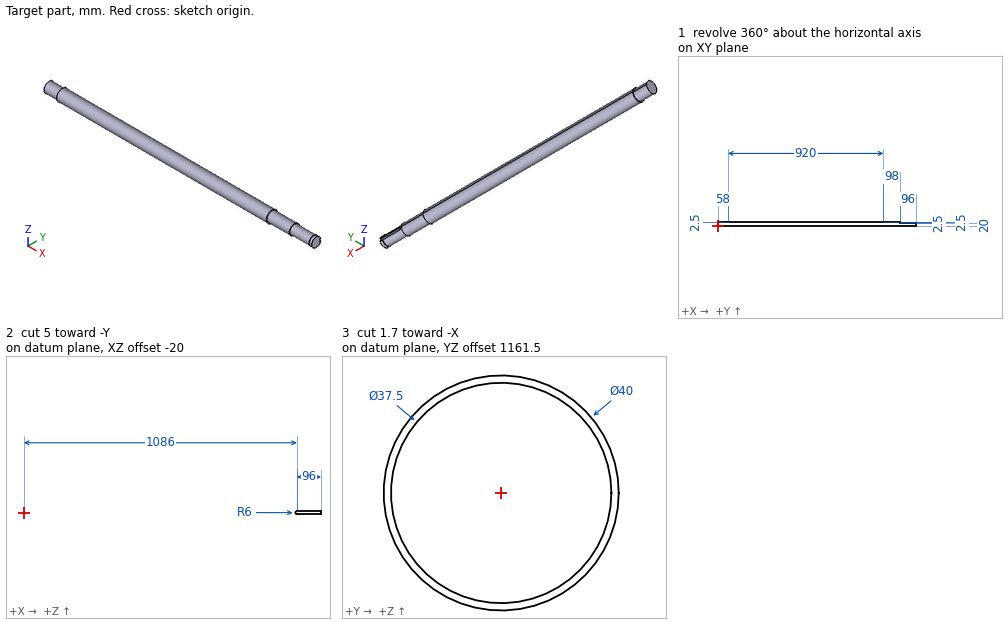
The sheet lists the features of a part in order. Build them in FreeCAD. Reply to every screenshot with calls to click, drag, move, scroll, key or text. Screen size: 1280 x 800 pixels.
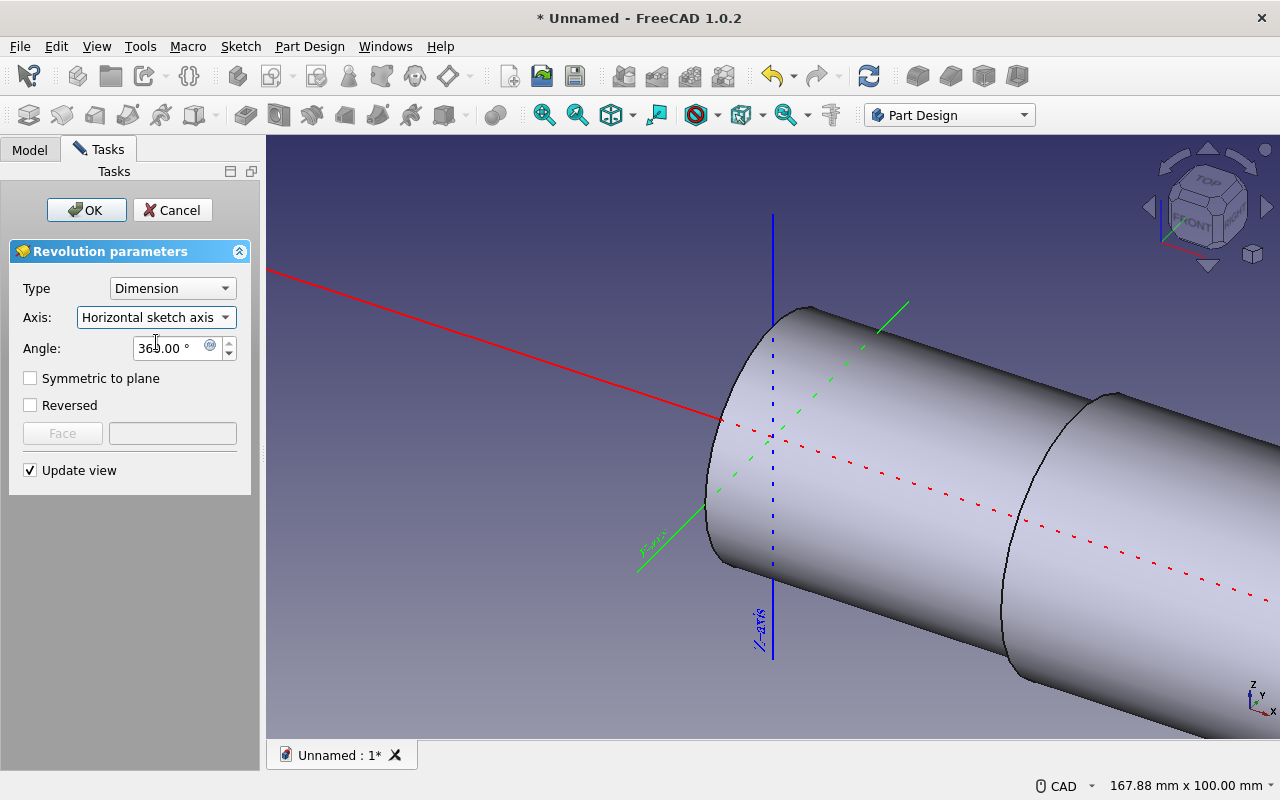
click(87, 210)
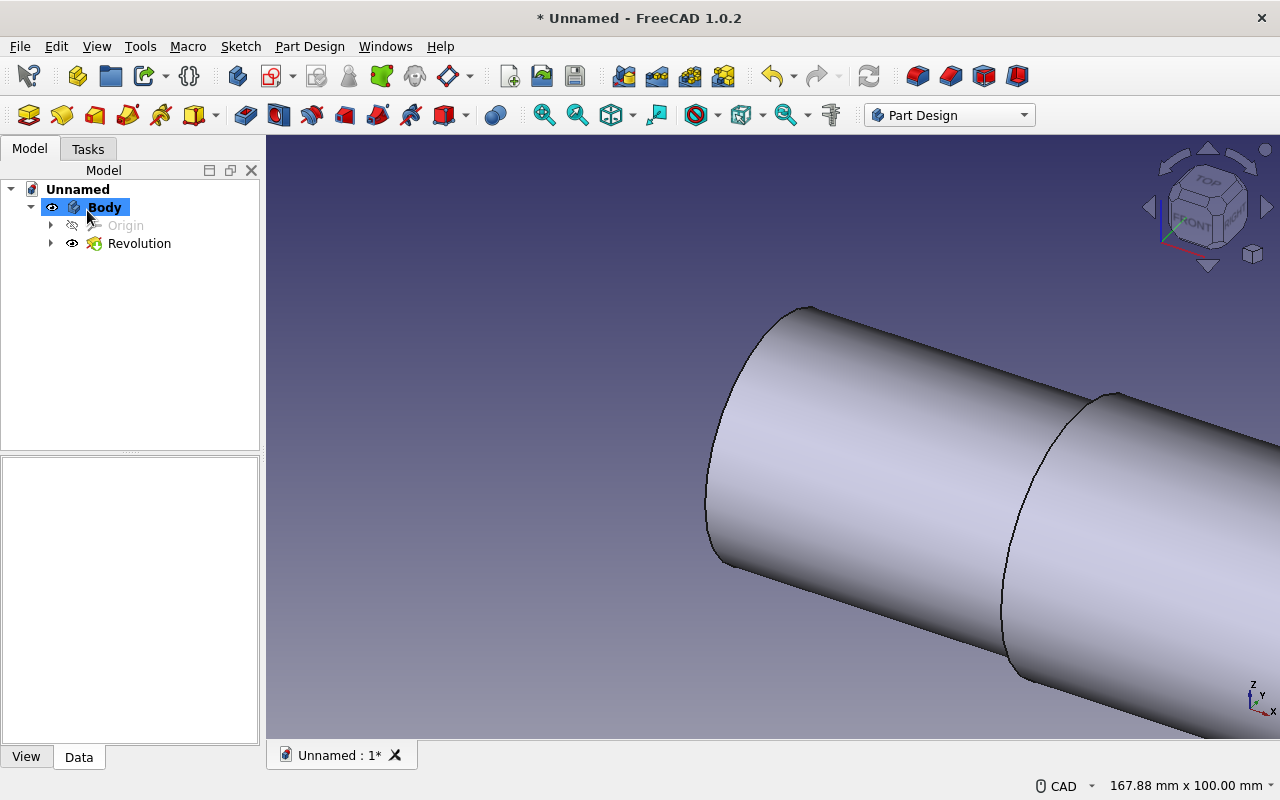
click(545, 116)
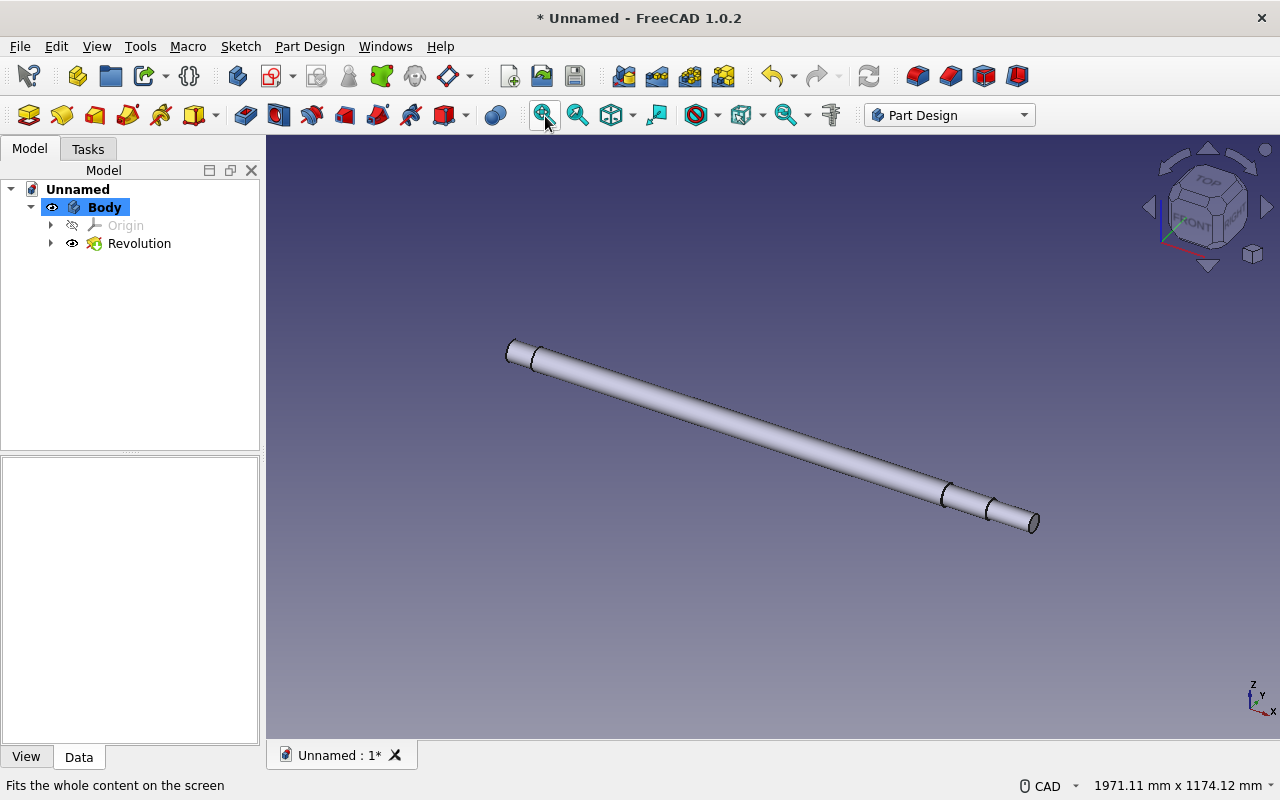
click(51, 225)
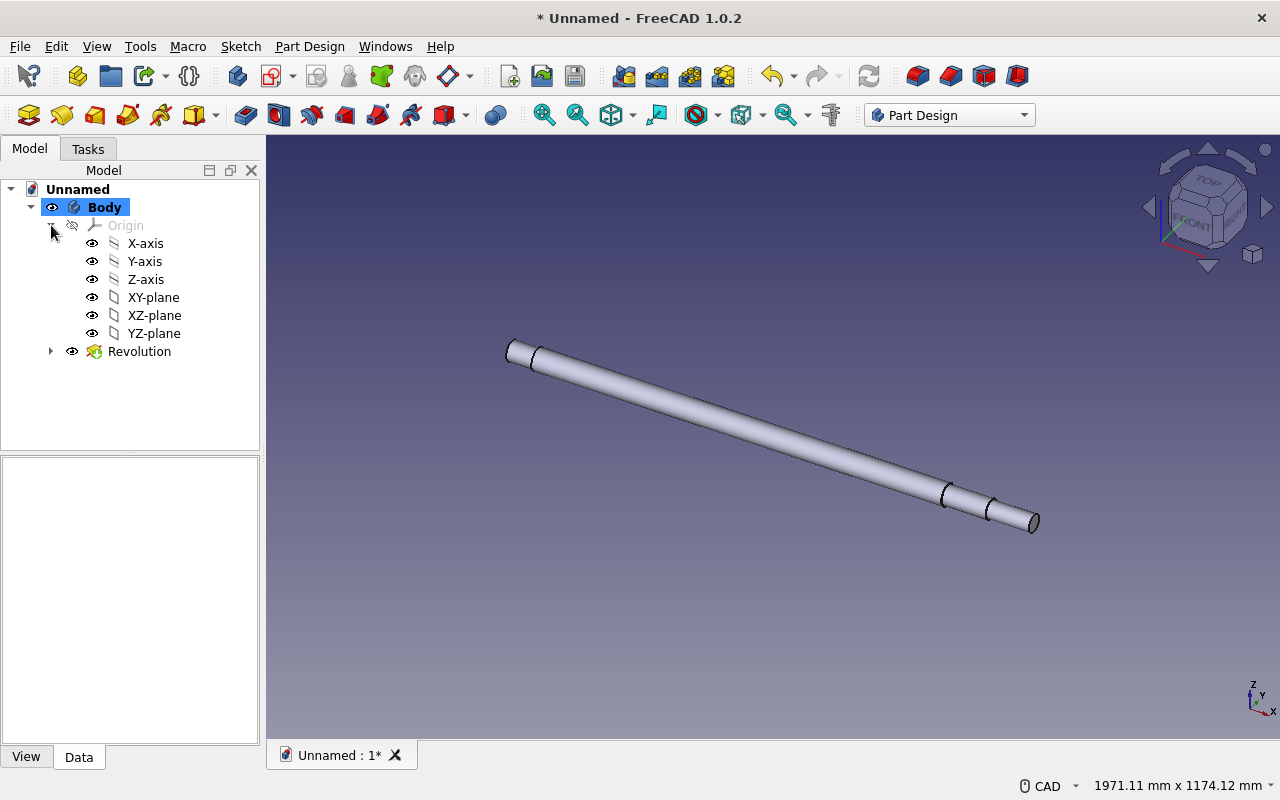
click(137, 315)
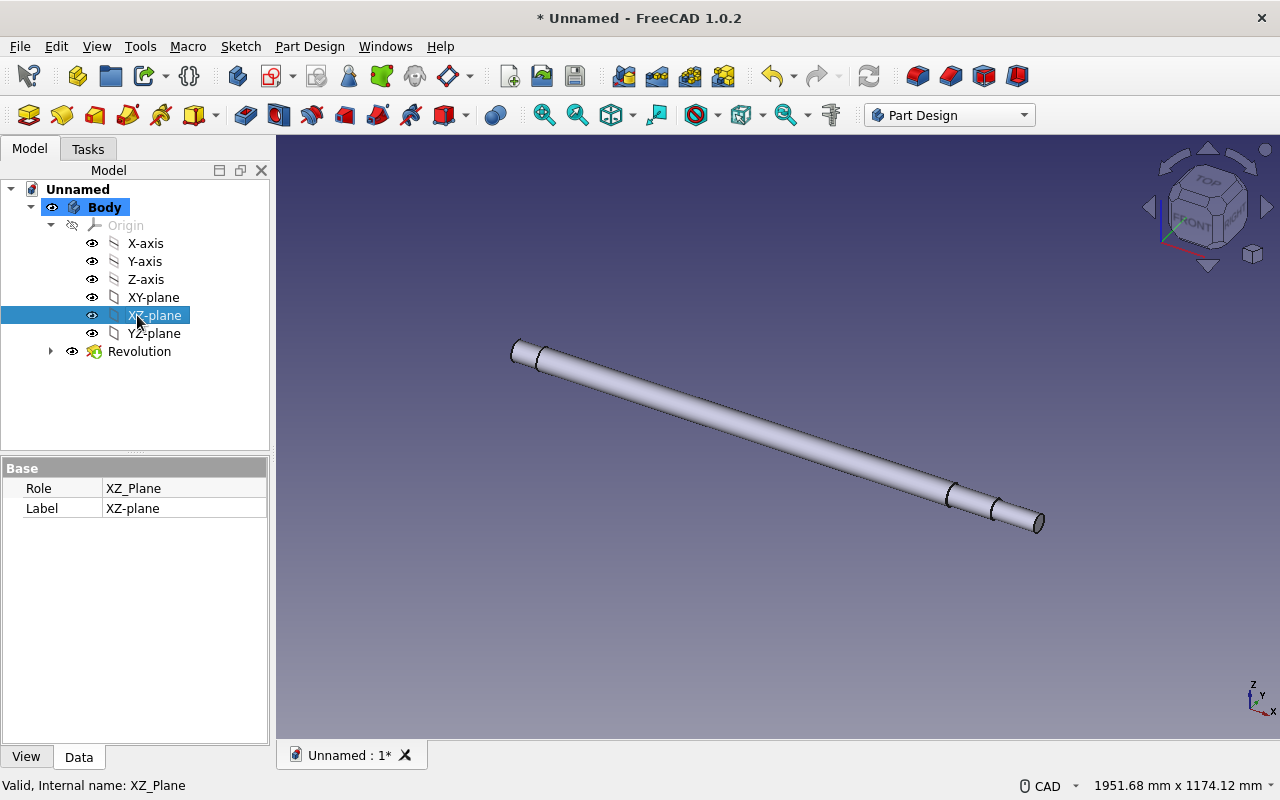
click(448, 76)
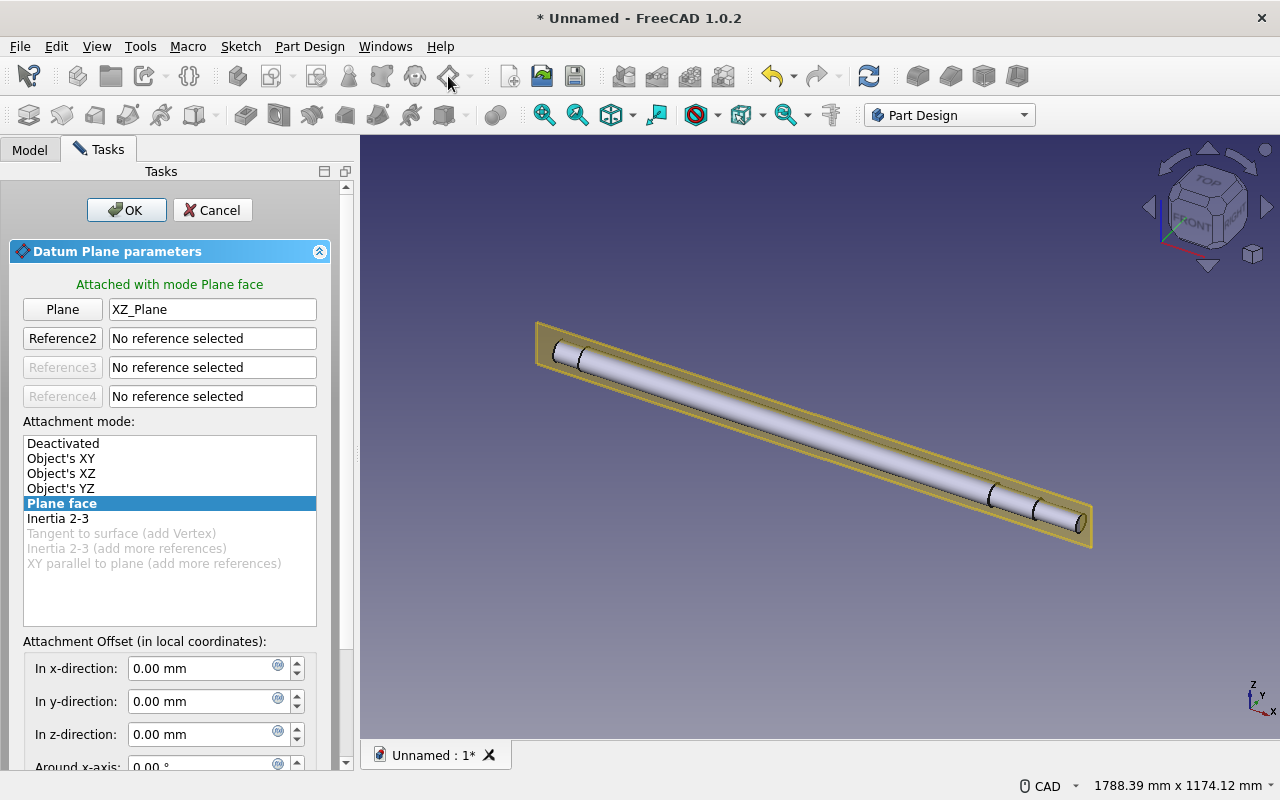
triple_click(210, 734)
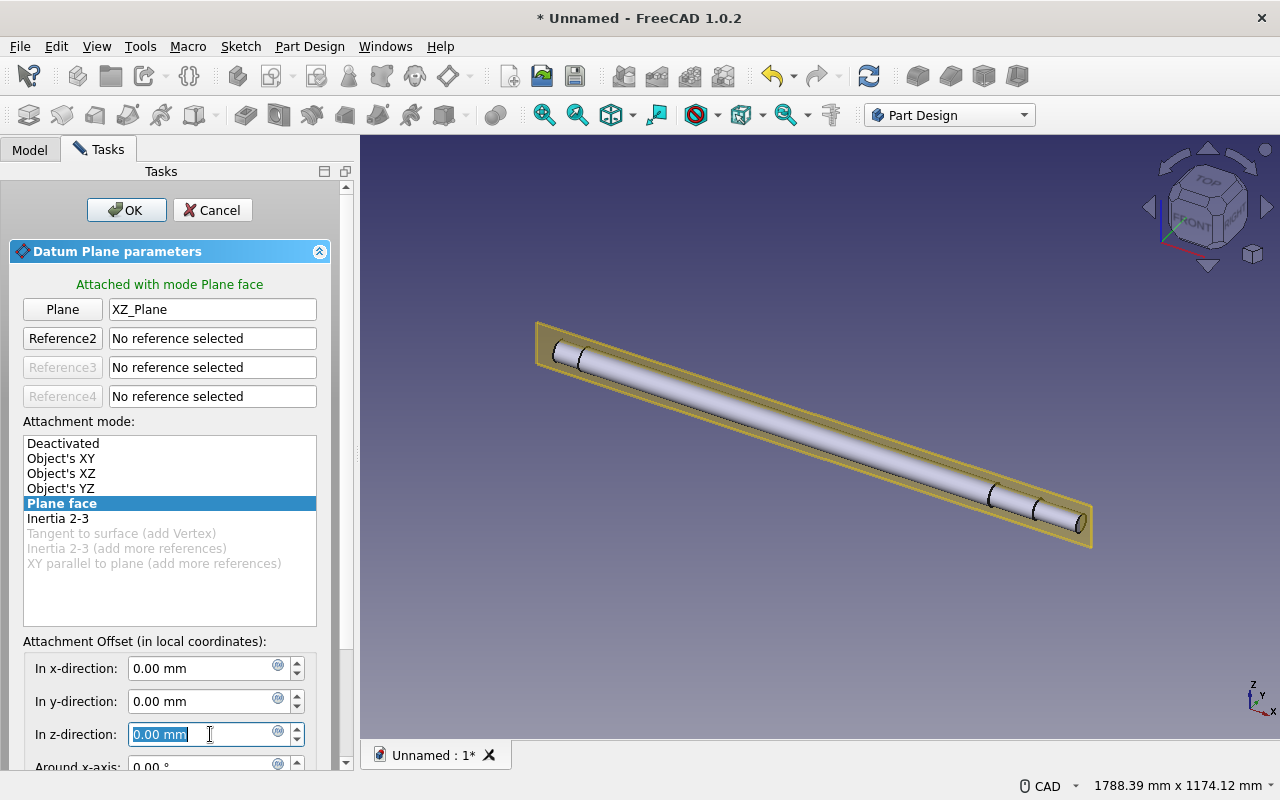
text(-20)
key(Tab)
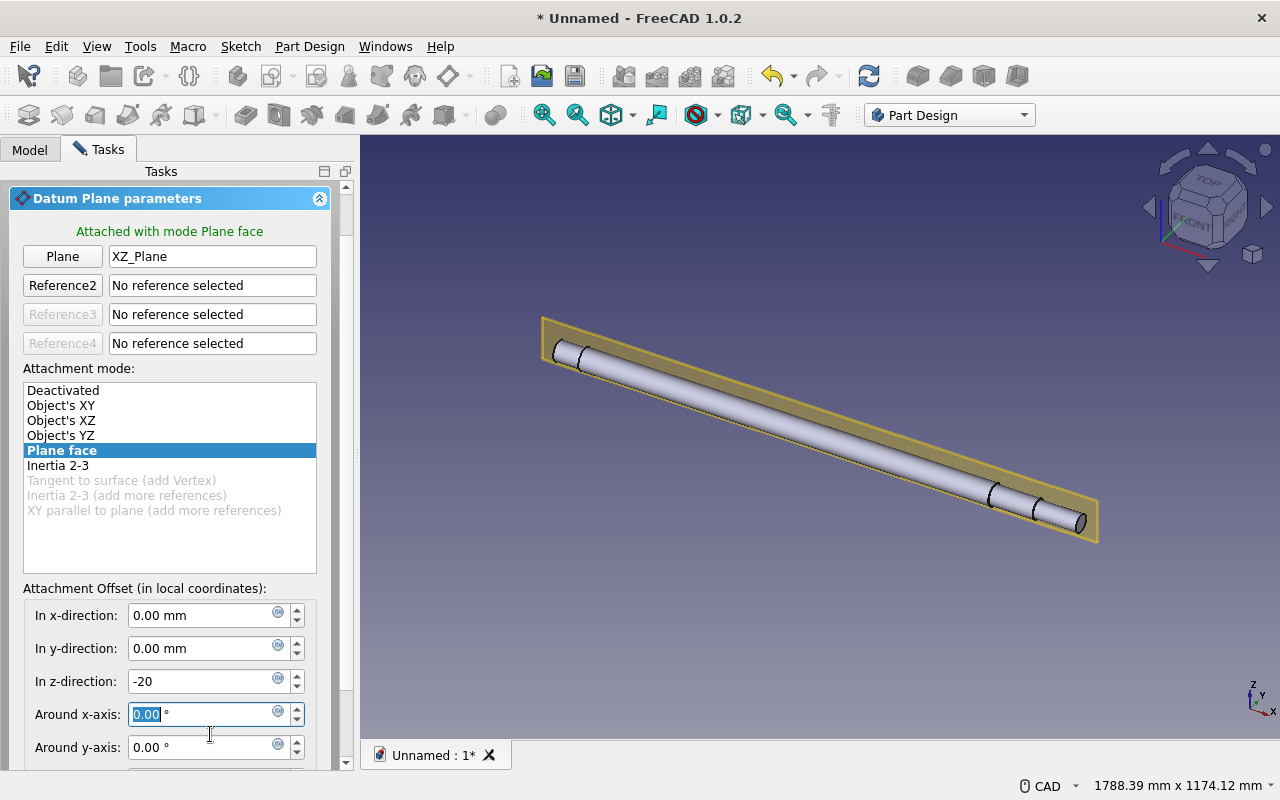
scroll(346, 476, up, 2)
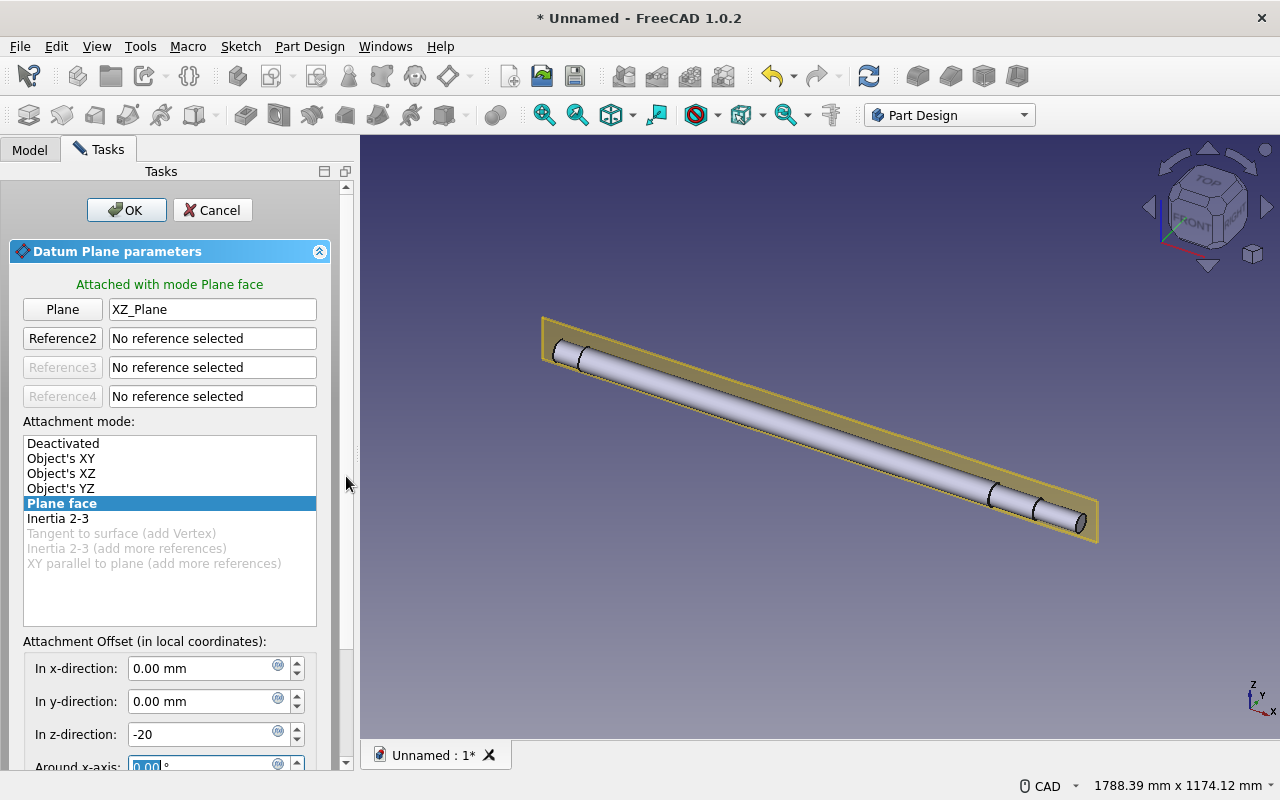
click(127, 210)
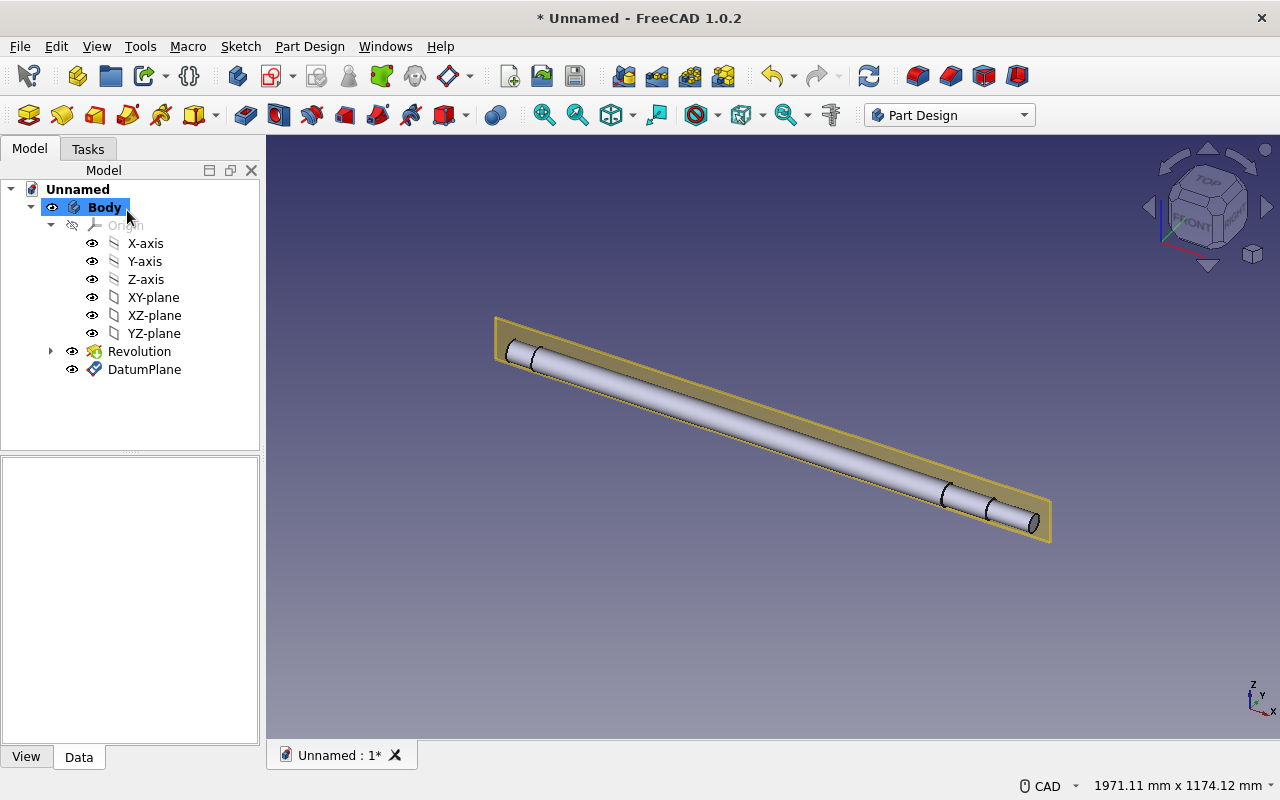
click(117, 369)